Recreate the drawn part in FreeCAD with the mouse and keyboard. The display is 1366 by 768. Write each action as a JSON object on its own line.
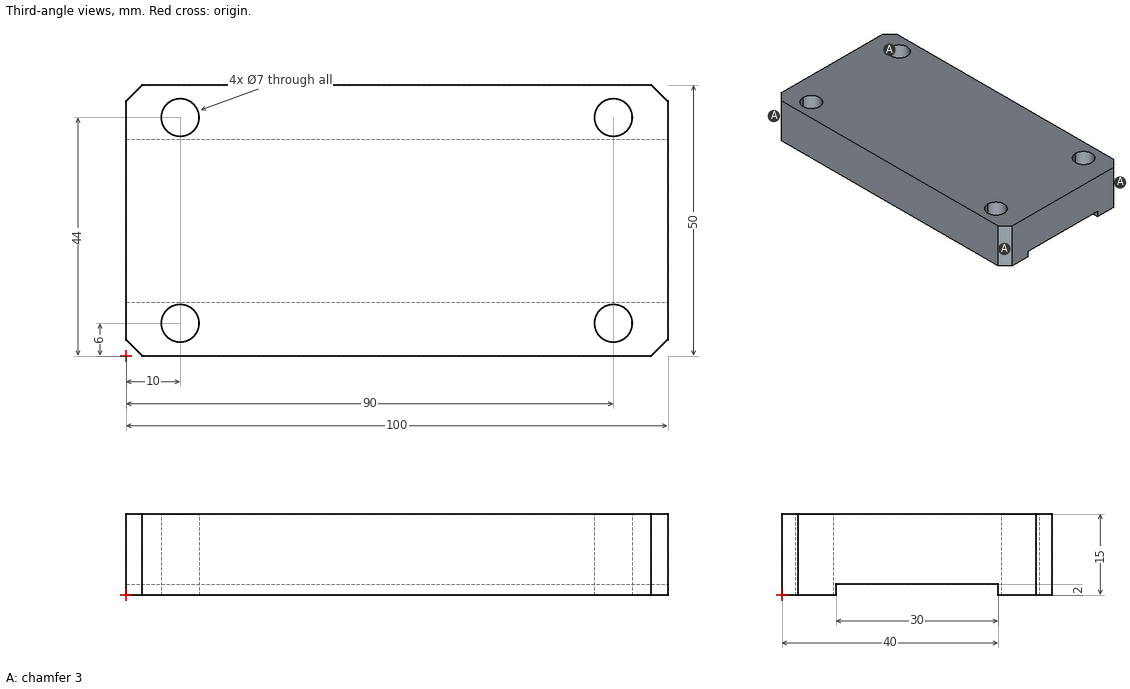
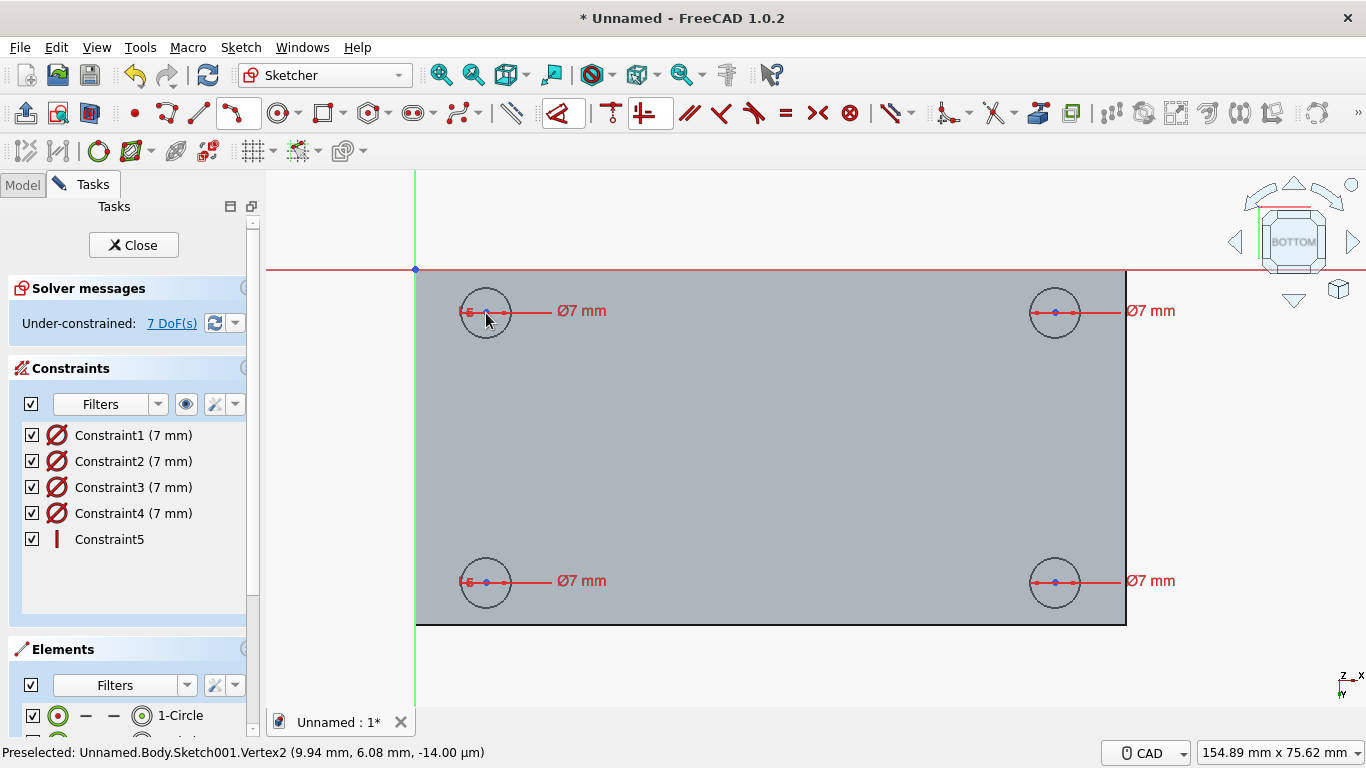
{"action": "left_click", "coordinate": [486, 583]}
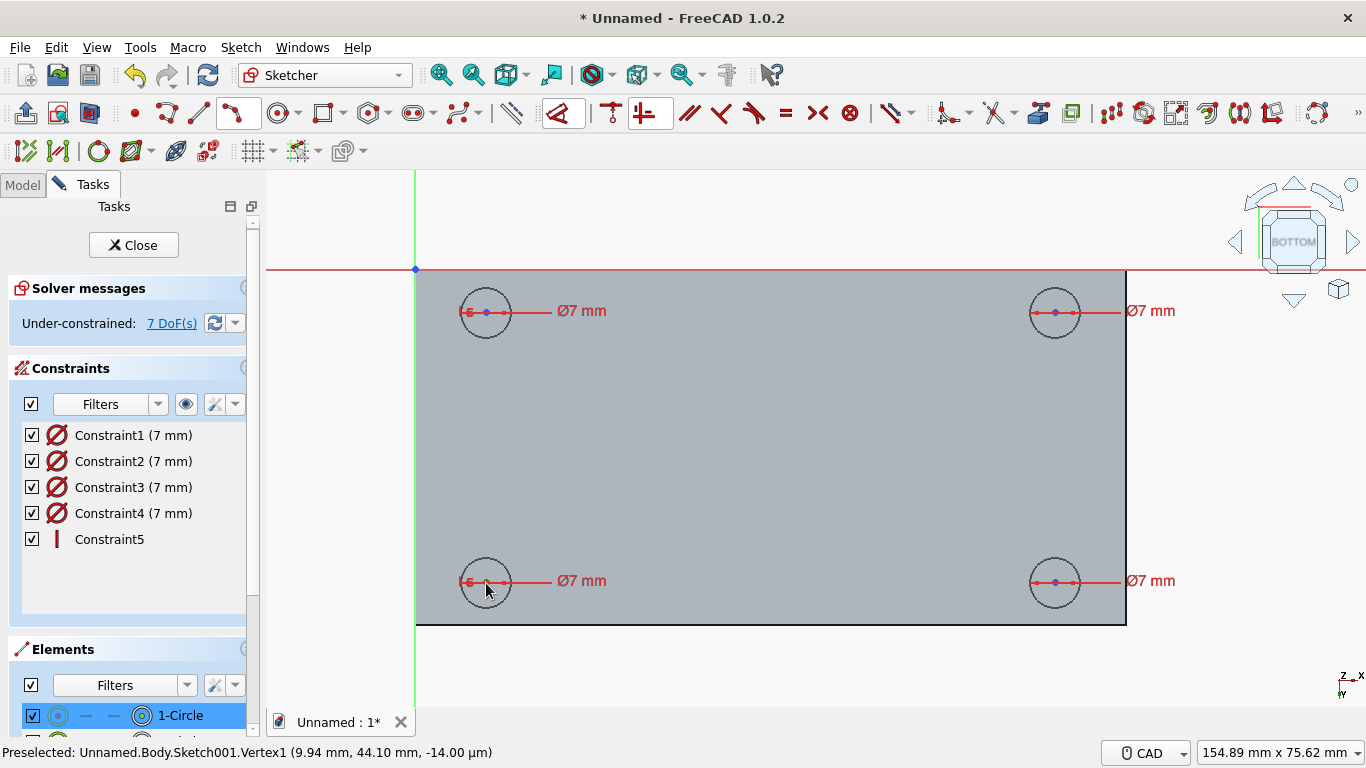
{"action": "left_click", "coordinate": [1055, 583]}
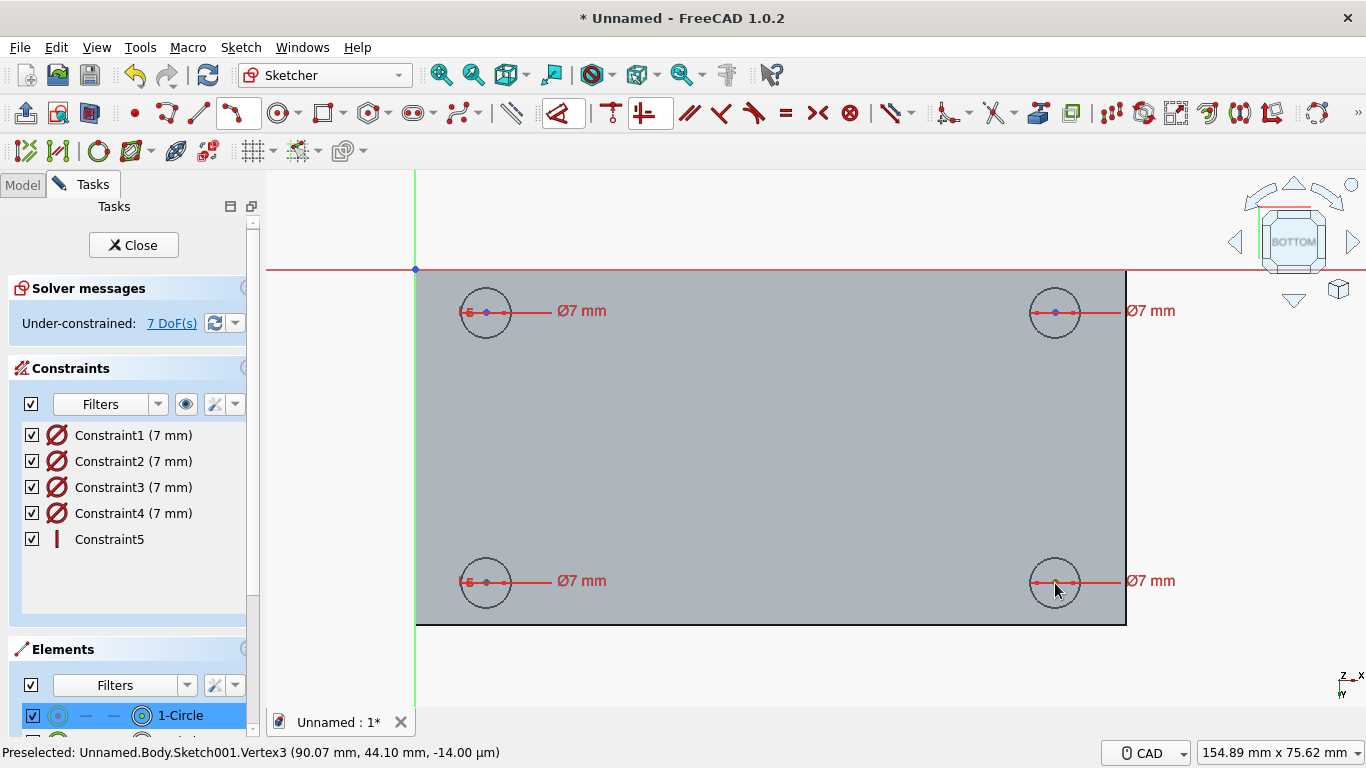
{"action": "left_click", "coordinate": [668, 114]}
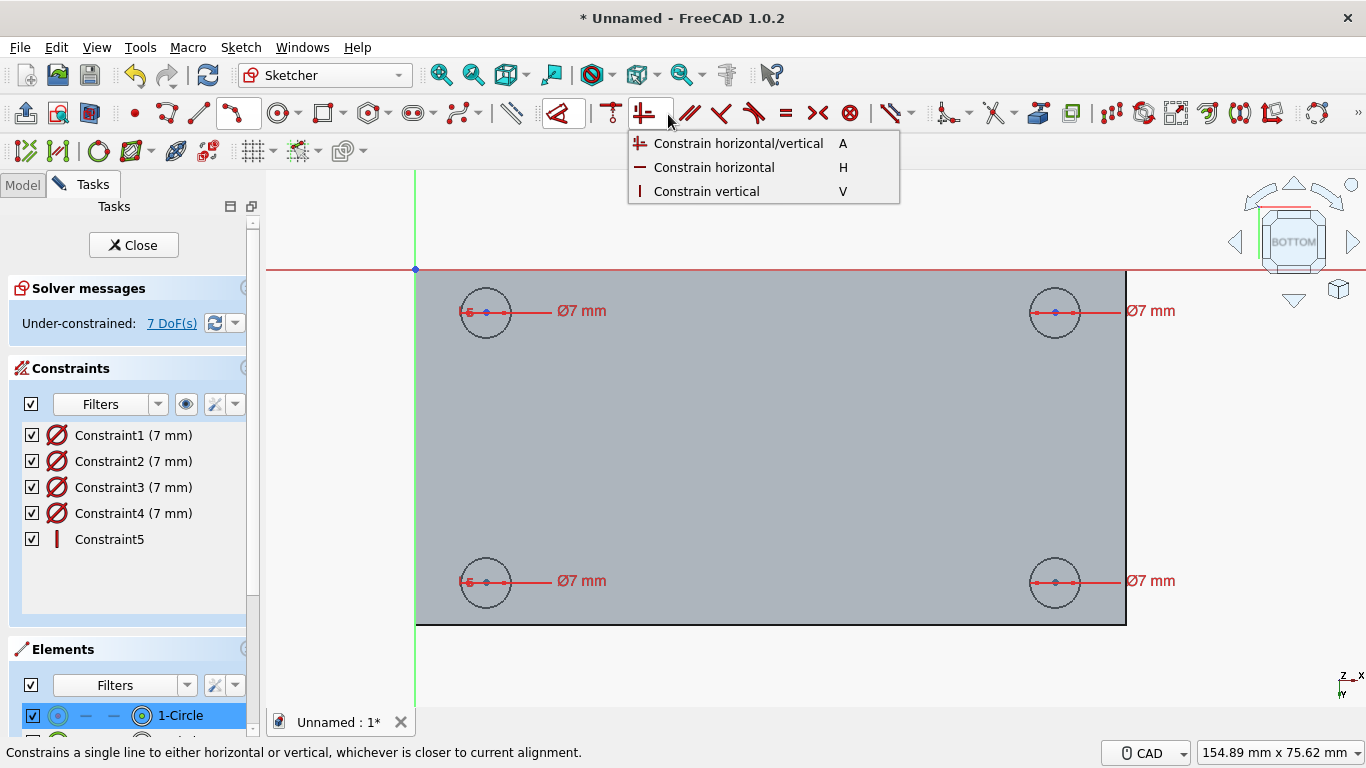
{"action": "left_click", "coordinate": [764, 167]}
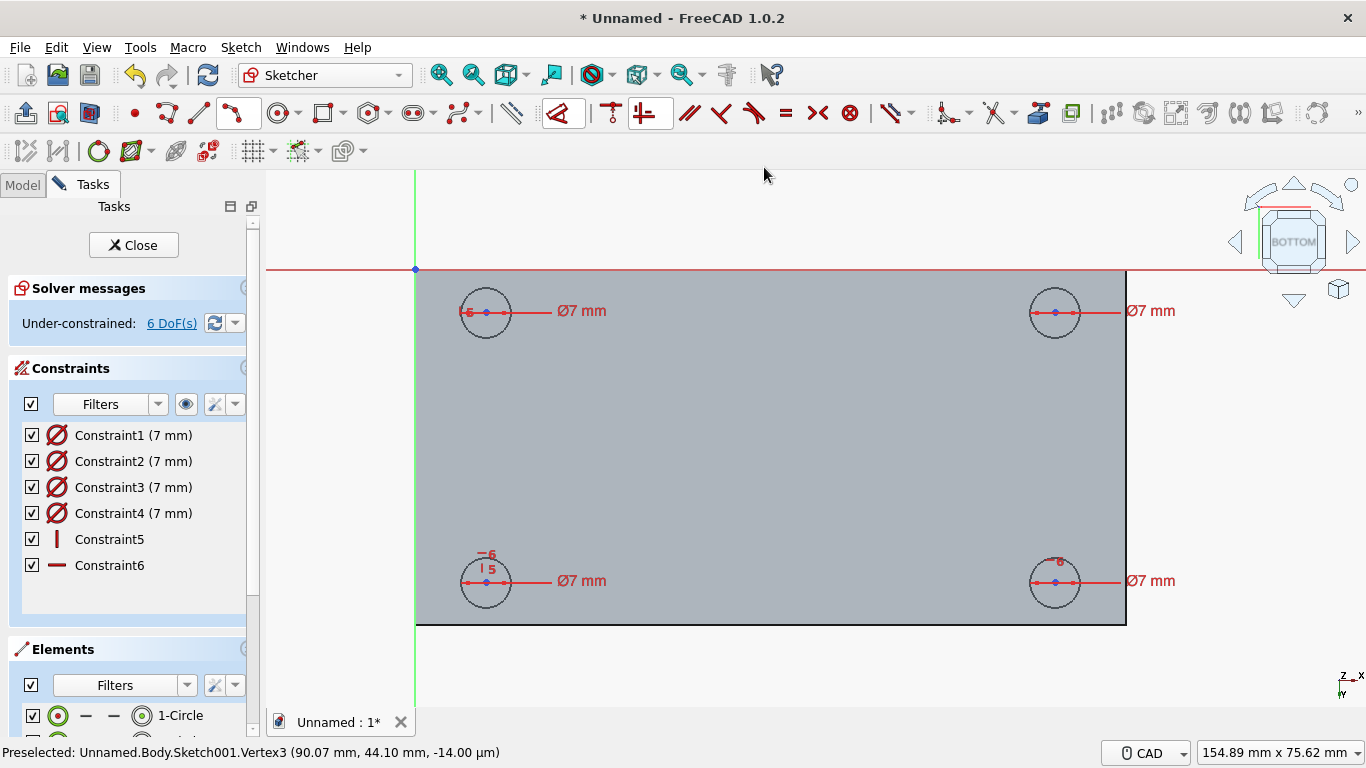
{"action": "left_click", "coordinate": [1055, 583]}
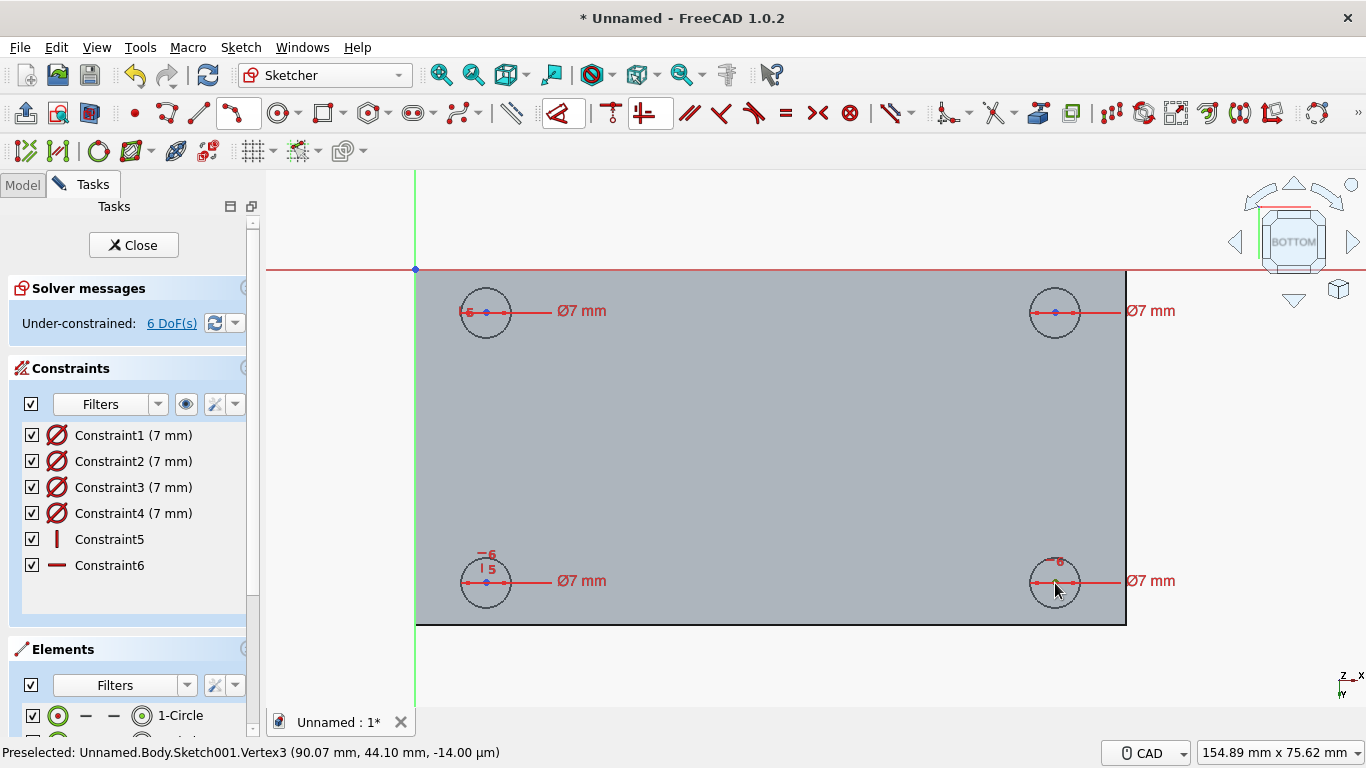
{"action": "left_click", "coordinate": [1055, 313]}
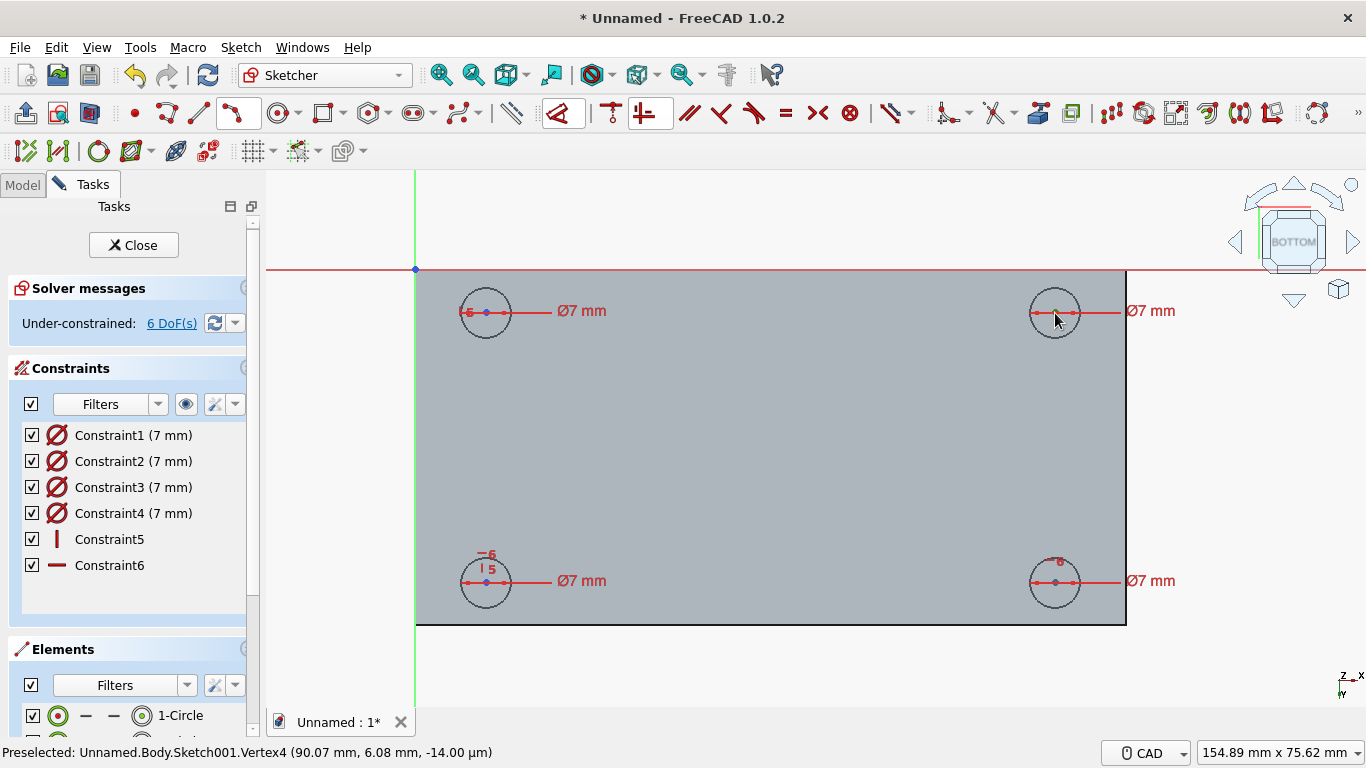
{"action": "key", "text": "v"}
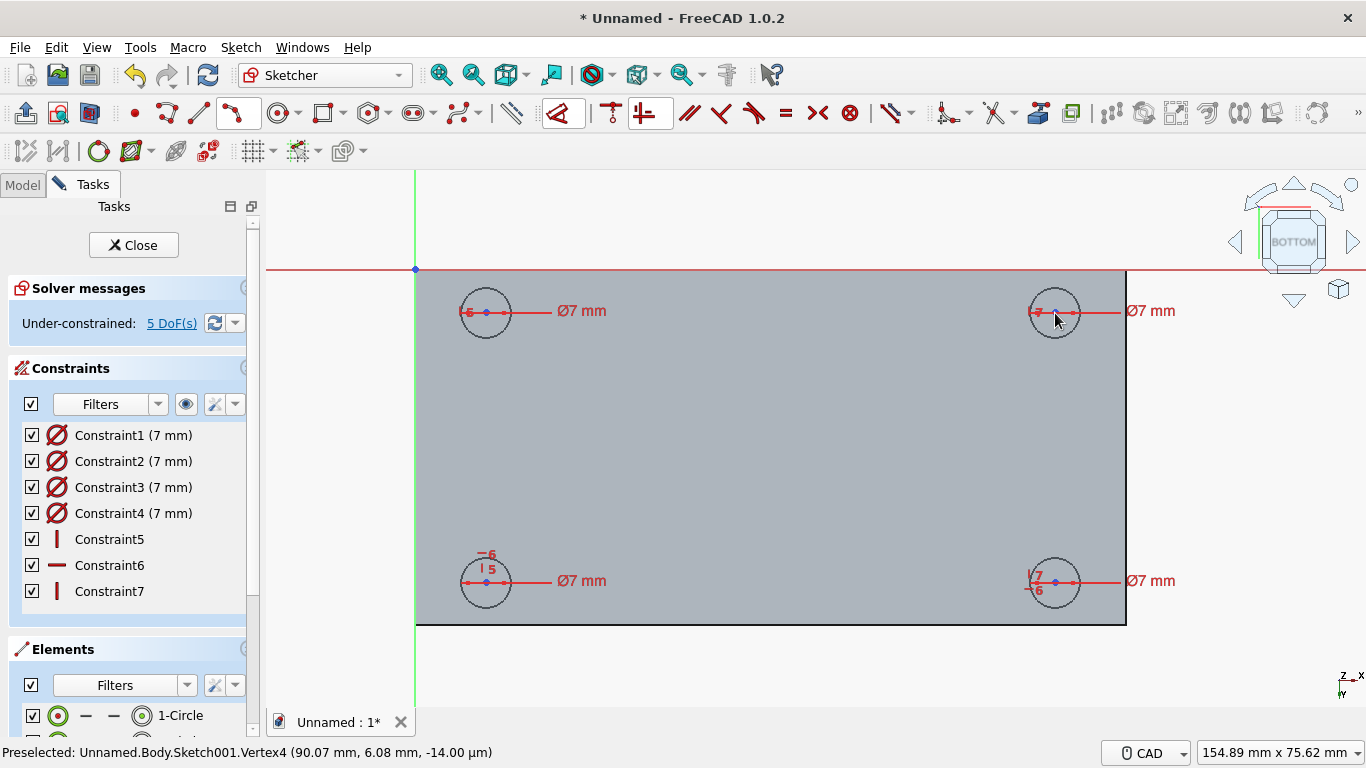
{"action": "left_click", "coordinate": [486, 313]}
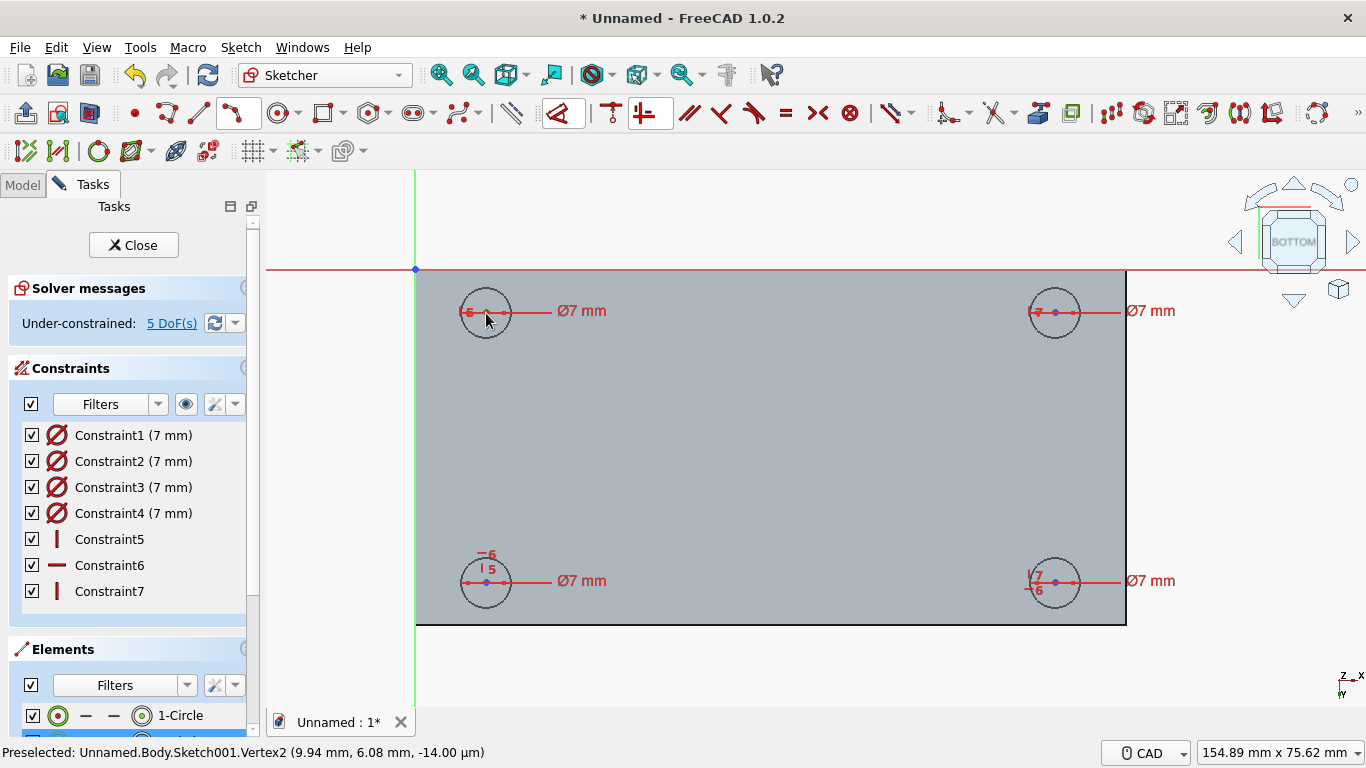
{"action": "left_click", "coordinate": [1055, 313]}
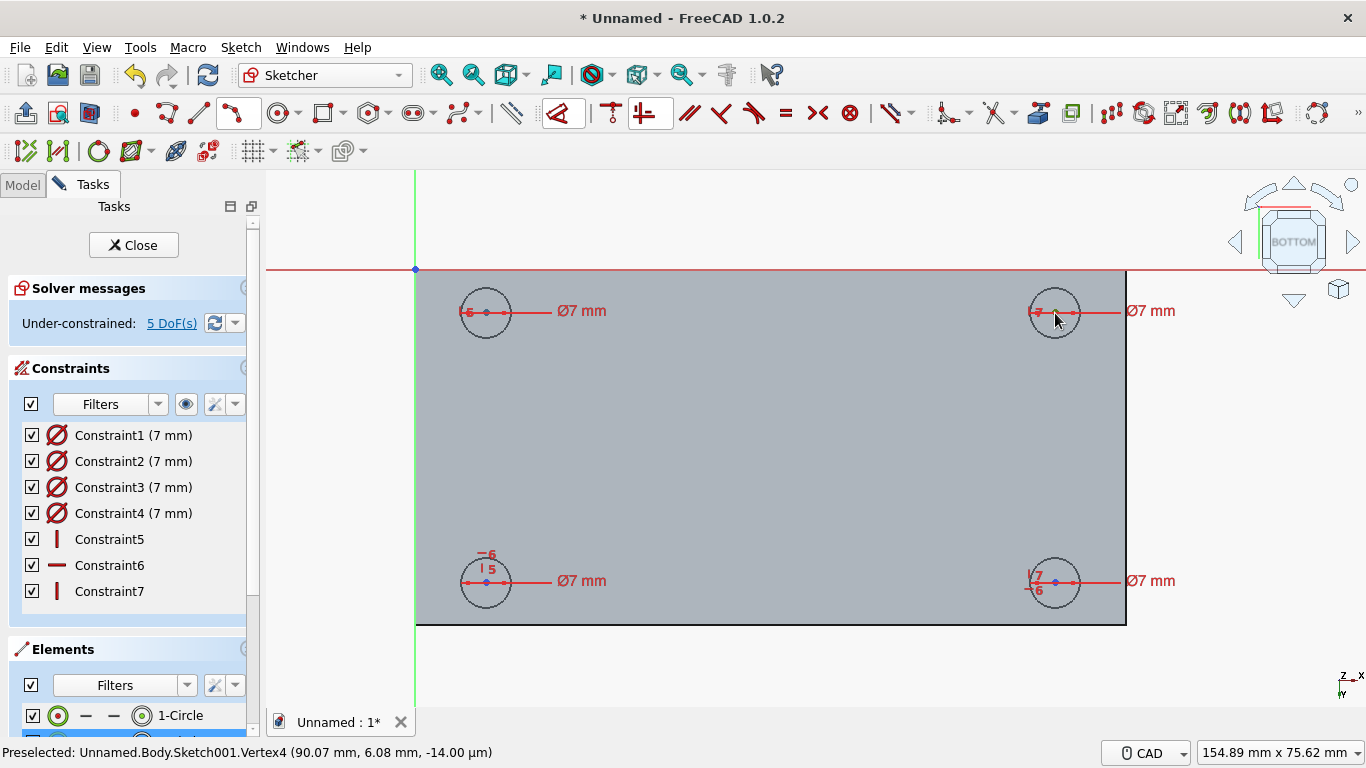
{"action": "key", "text": "h"}